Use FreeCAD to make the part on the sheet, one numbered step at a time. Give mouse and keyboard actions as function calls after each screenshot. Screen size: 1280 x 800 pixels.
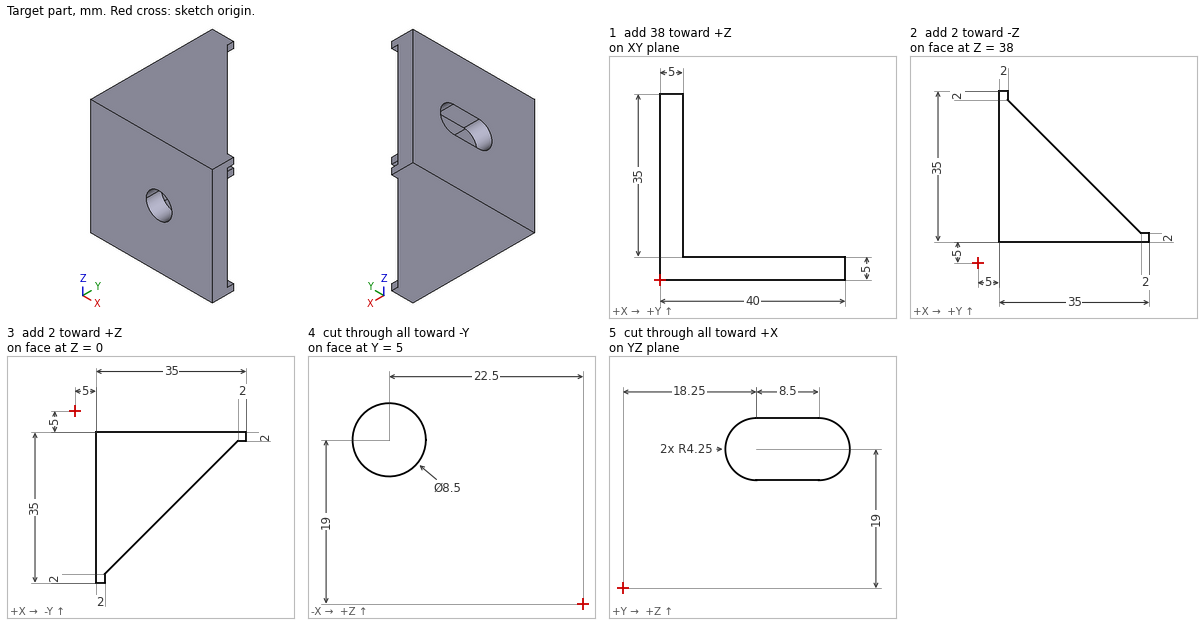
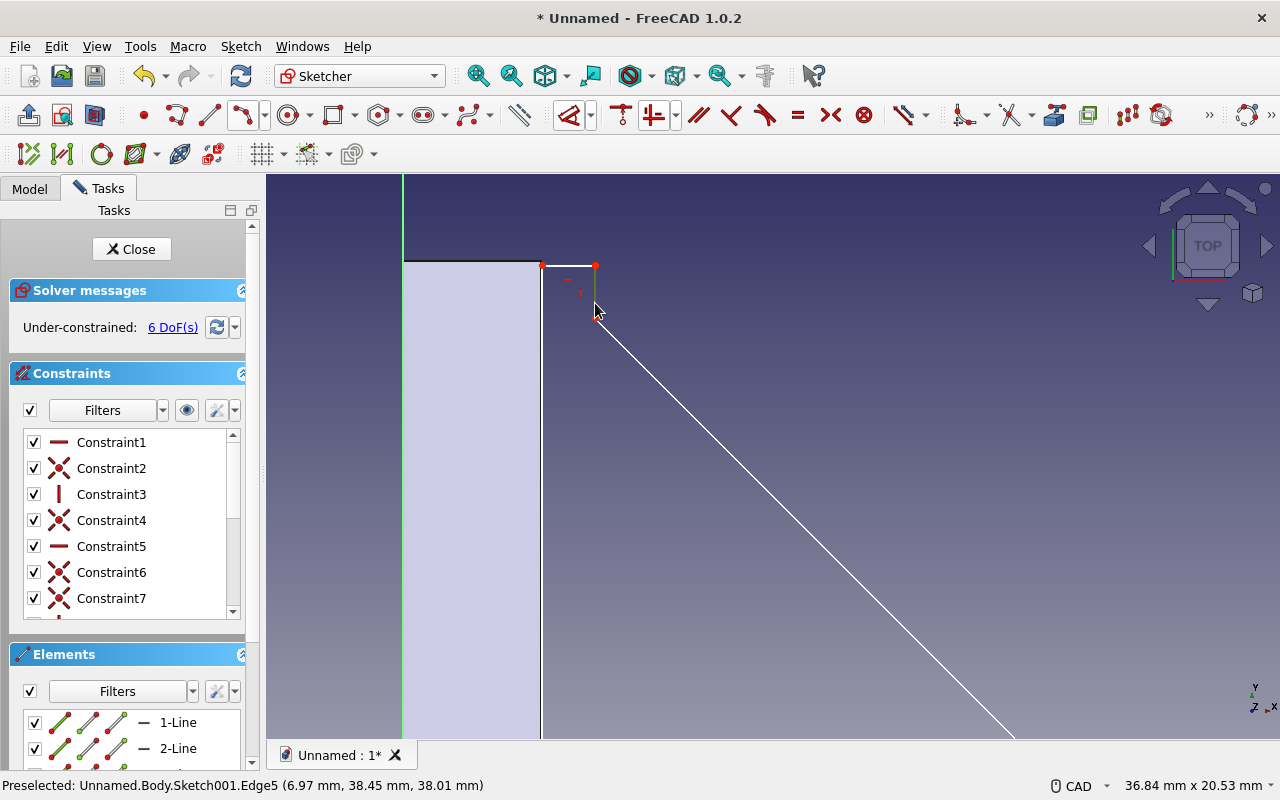
click(590, 116)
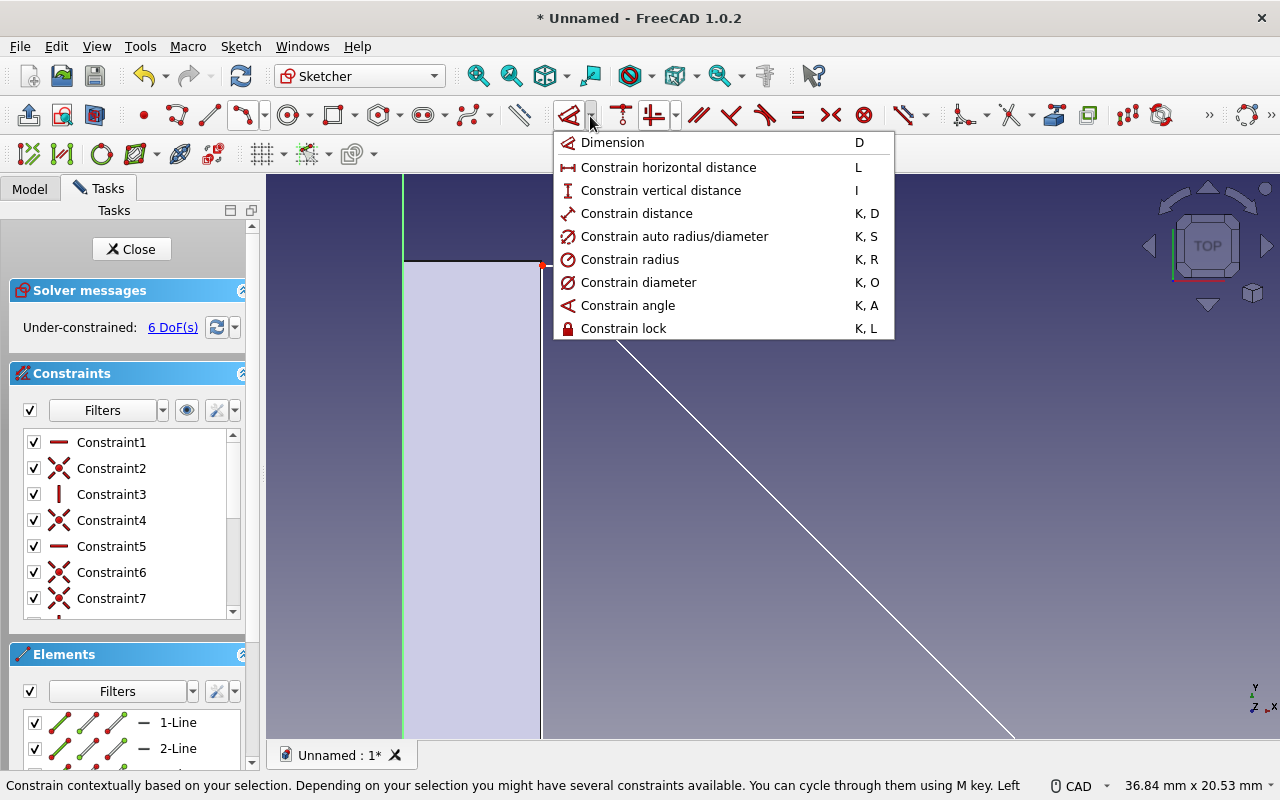
click(724, 190)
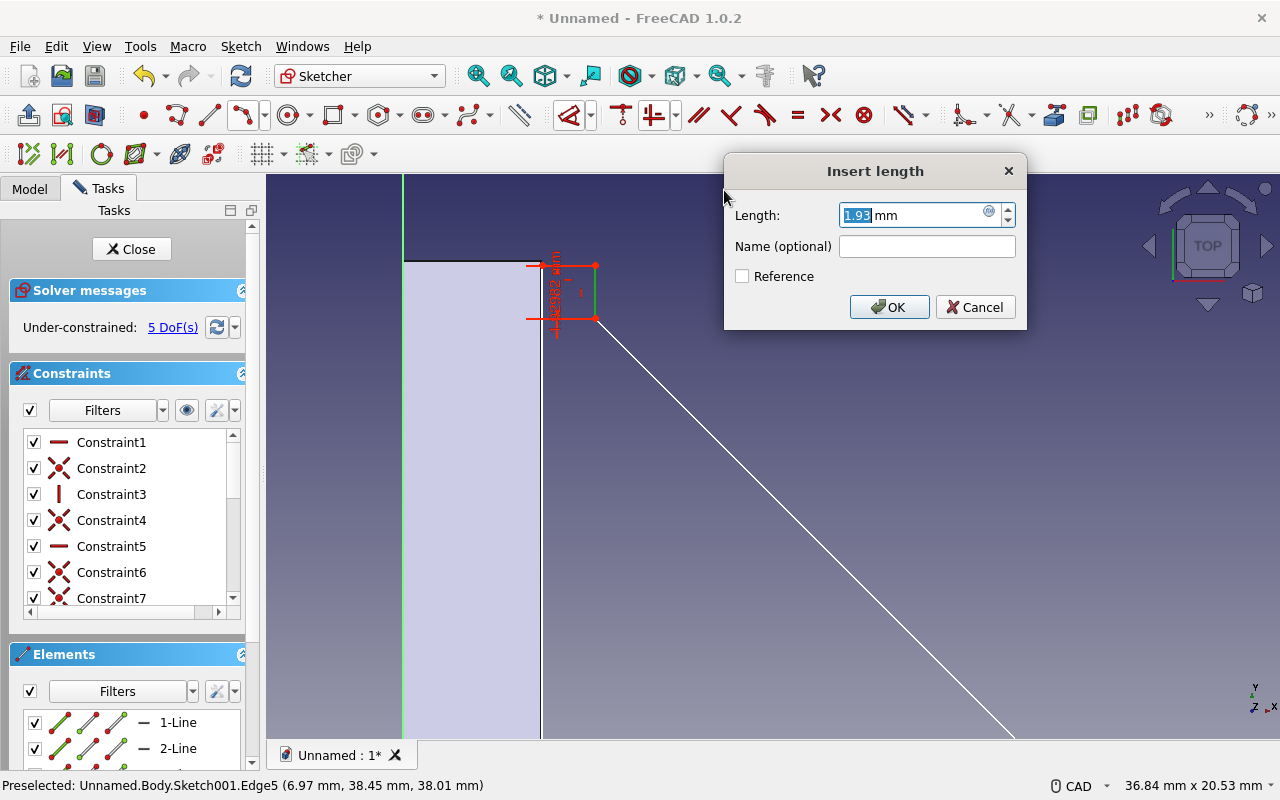
text(2)
key(Return)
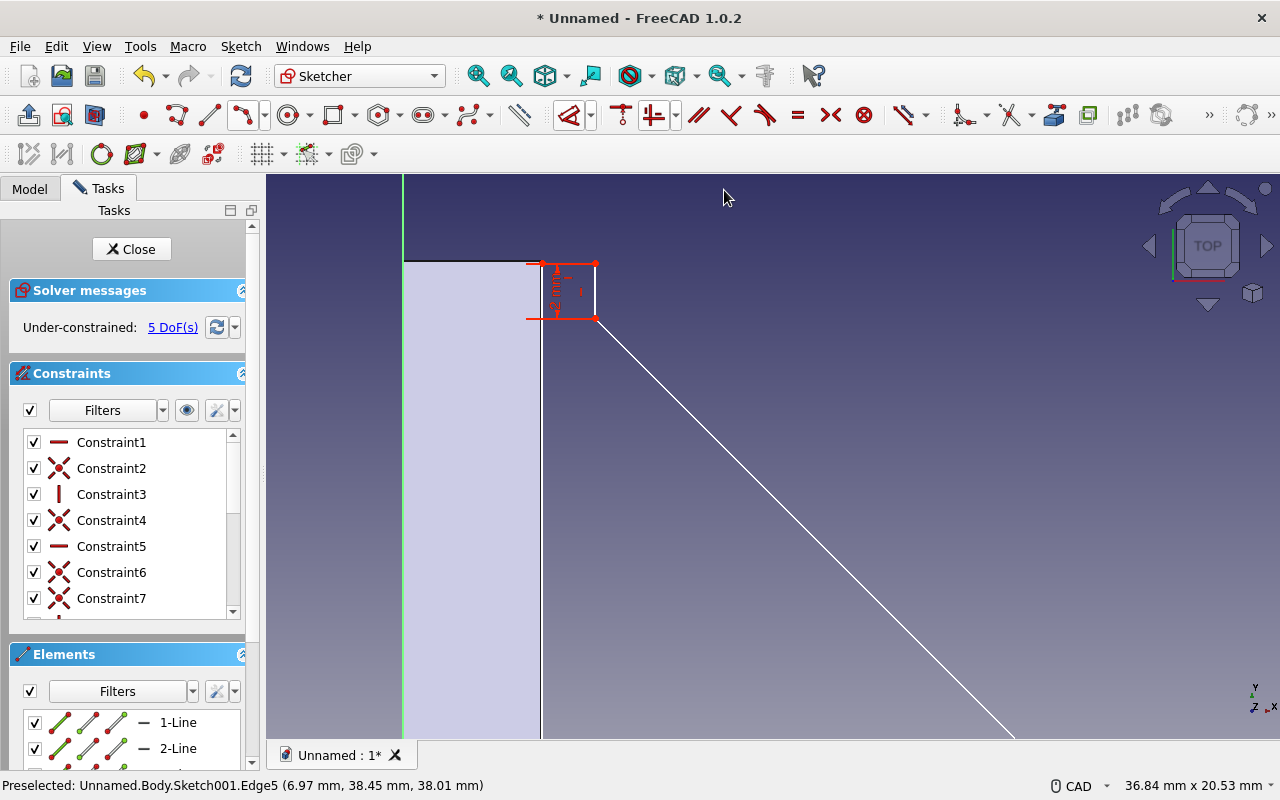
click(579, 264)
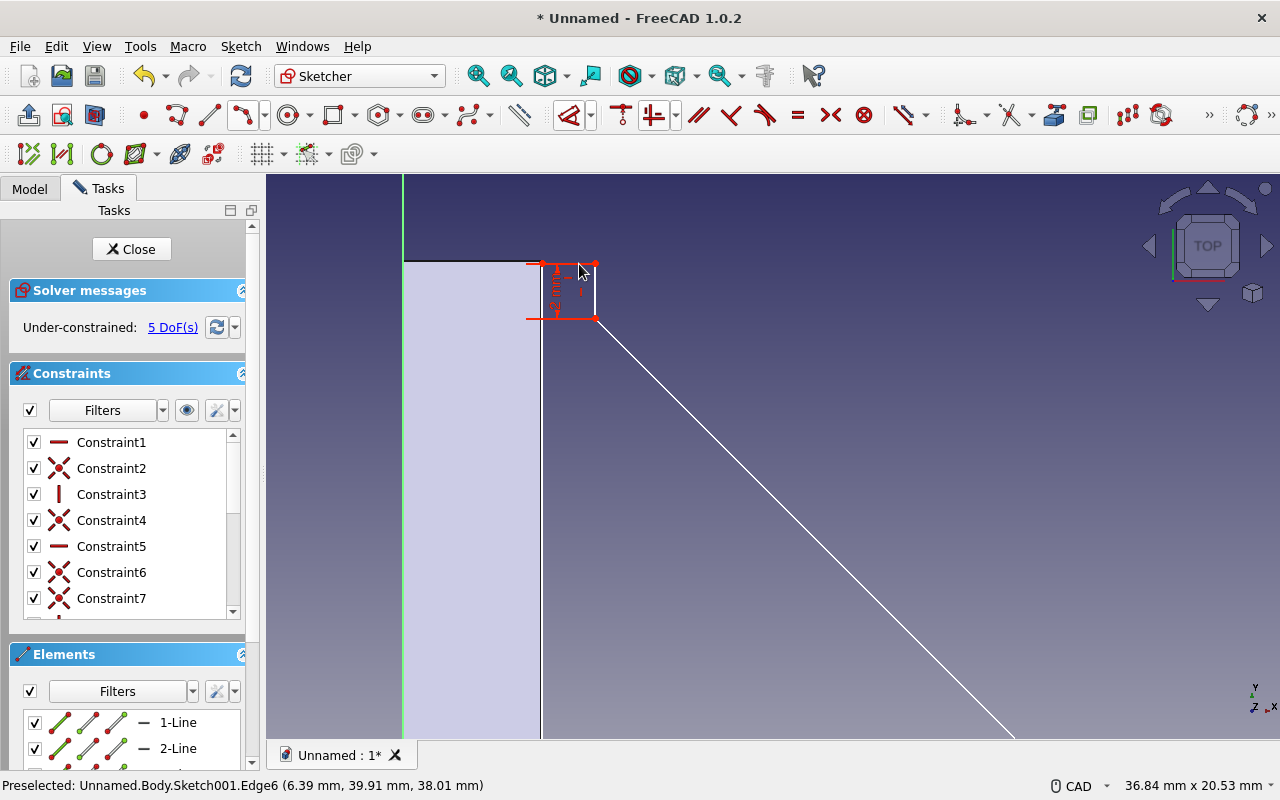
click(590, 116)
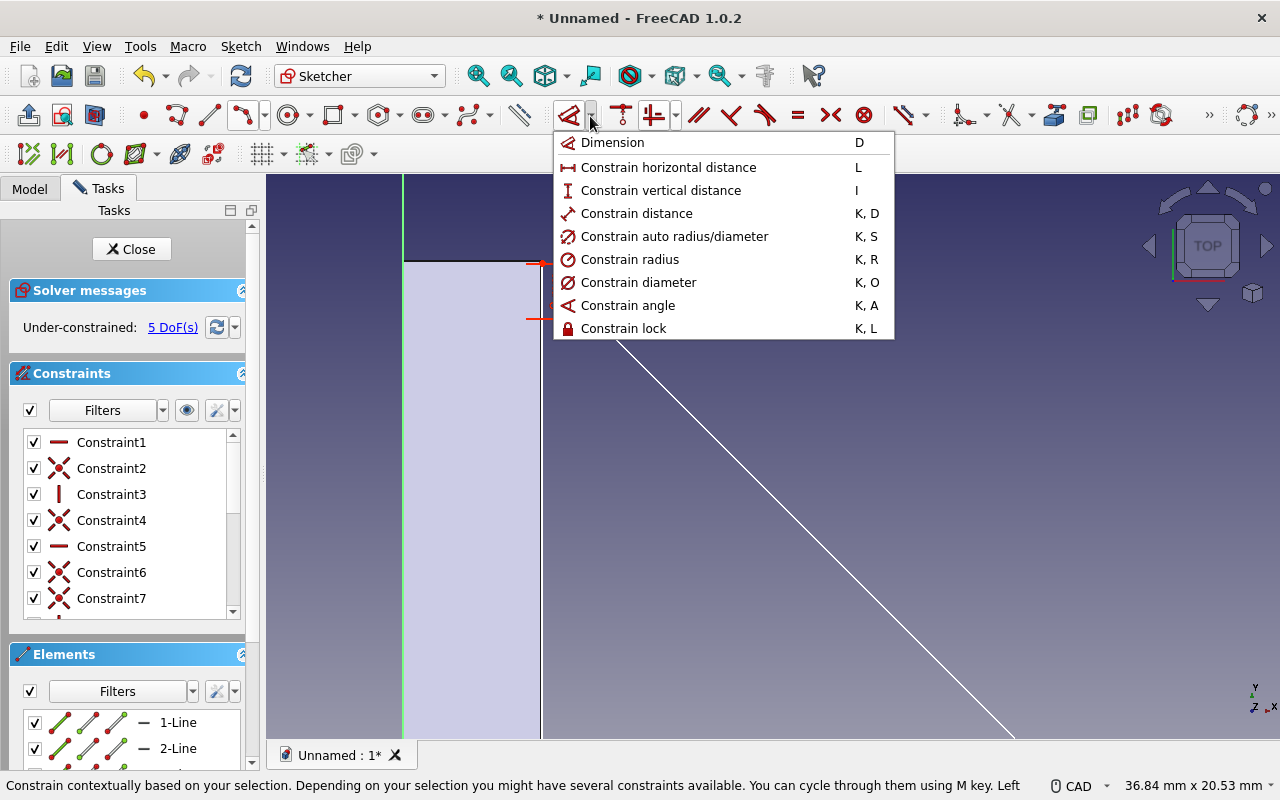
click(724, 168)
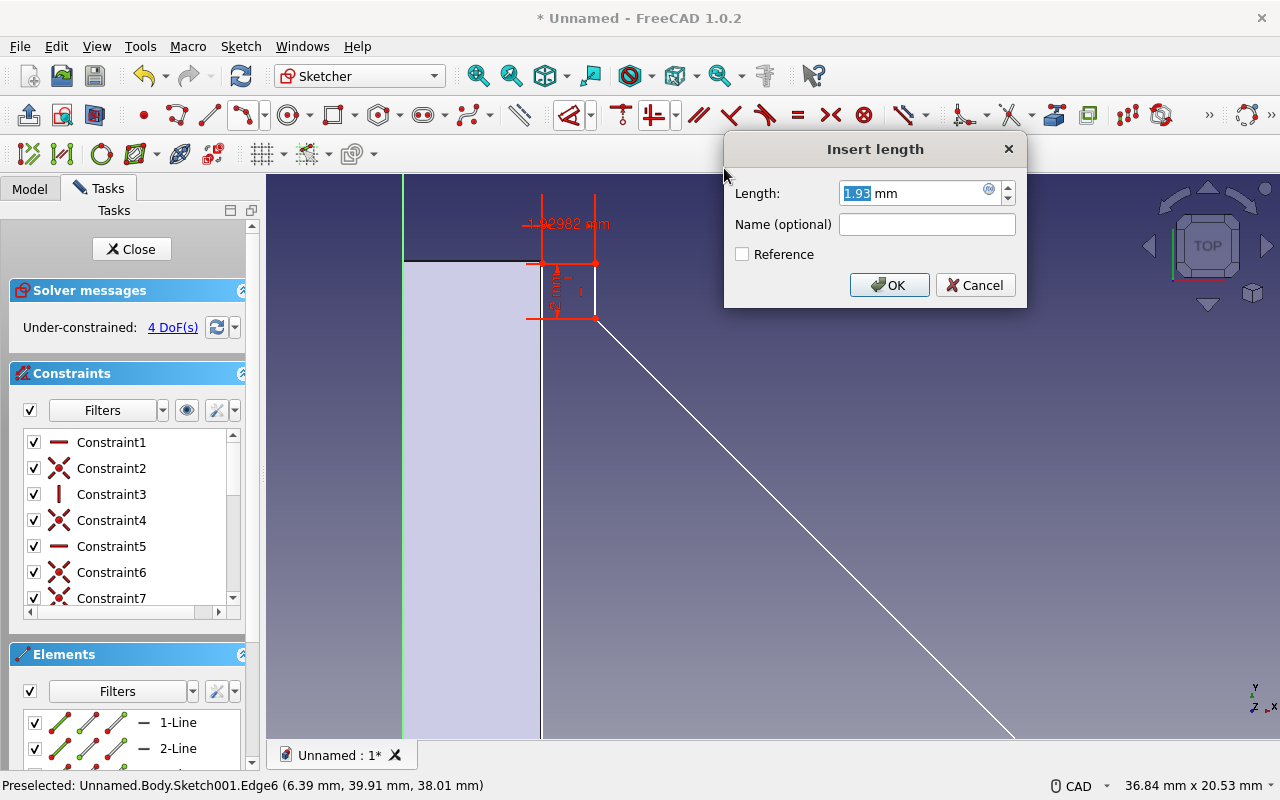
text(2)
key(Return)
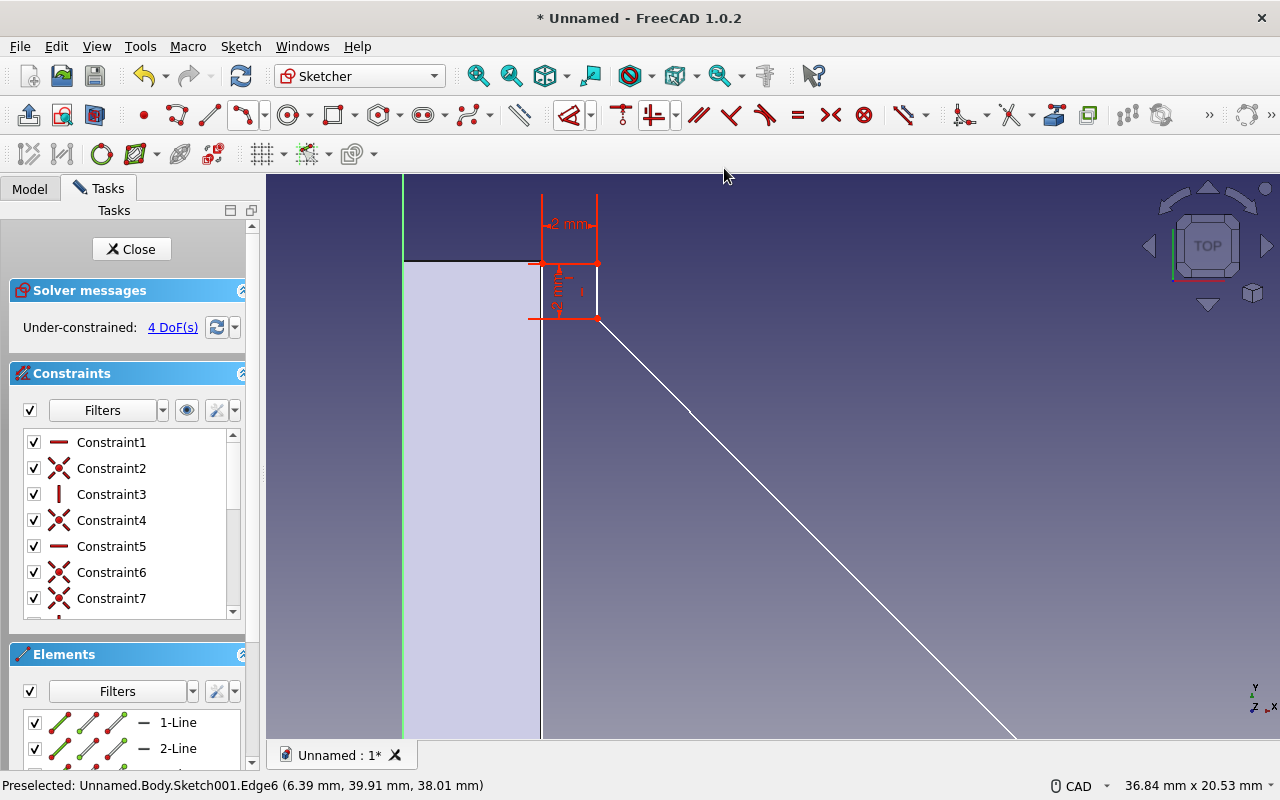
scroll(597, 303, down, 6)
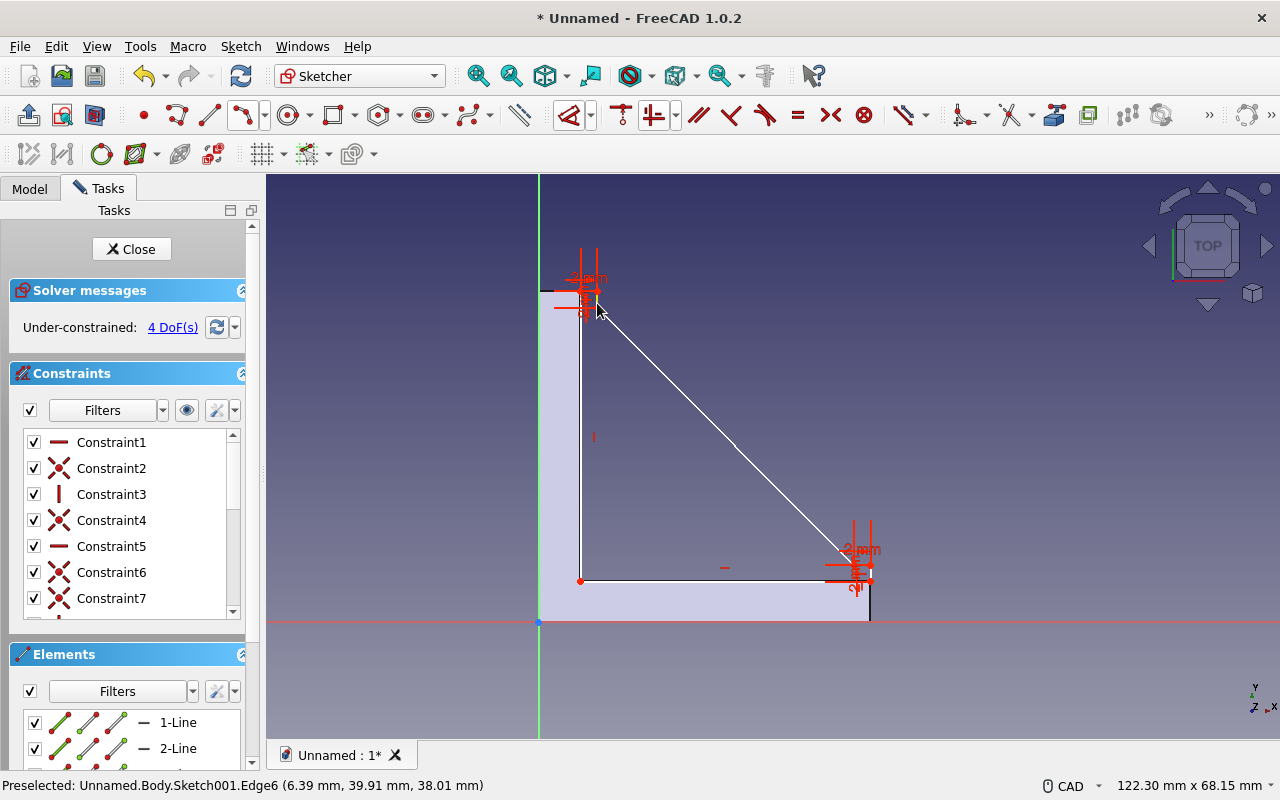
click(668, 582)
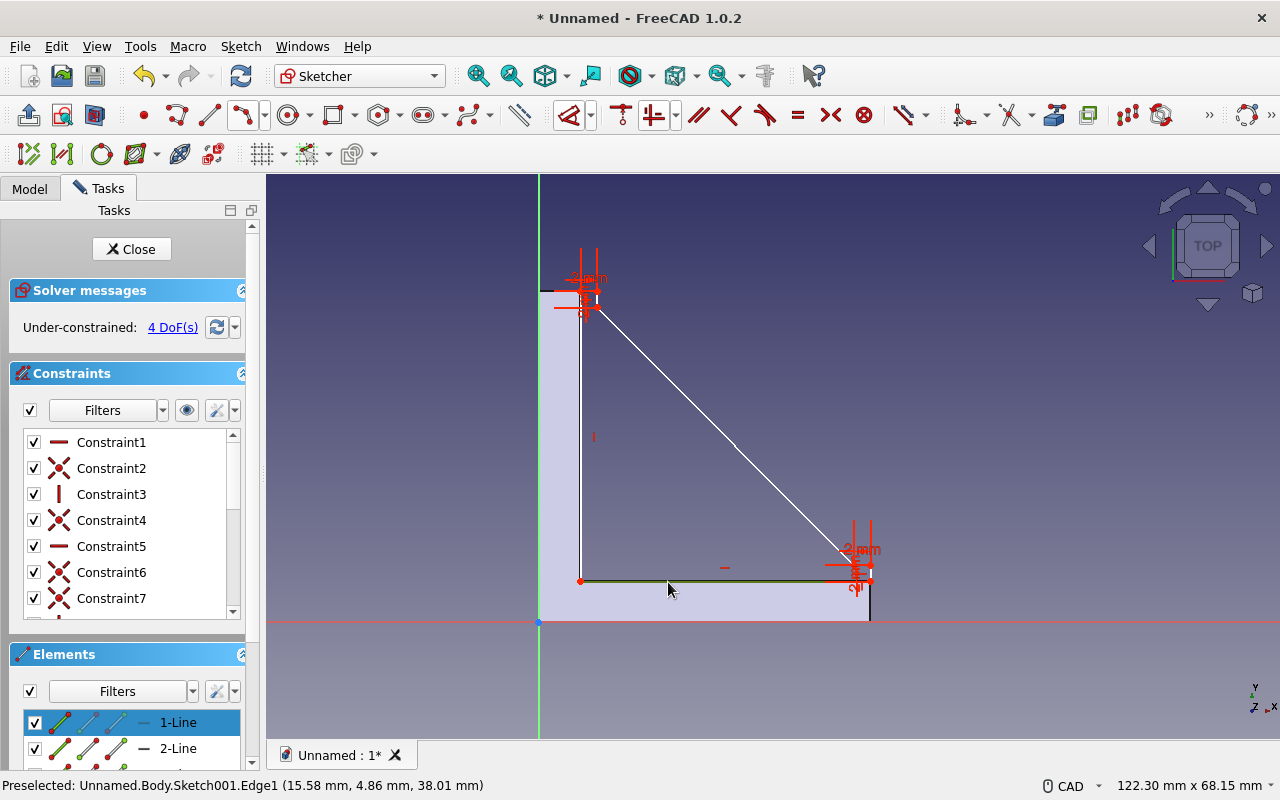
key(l)